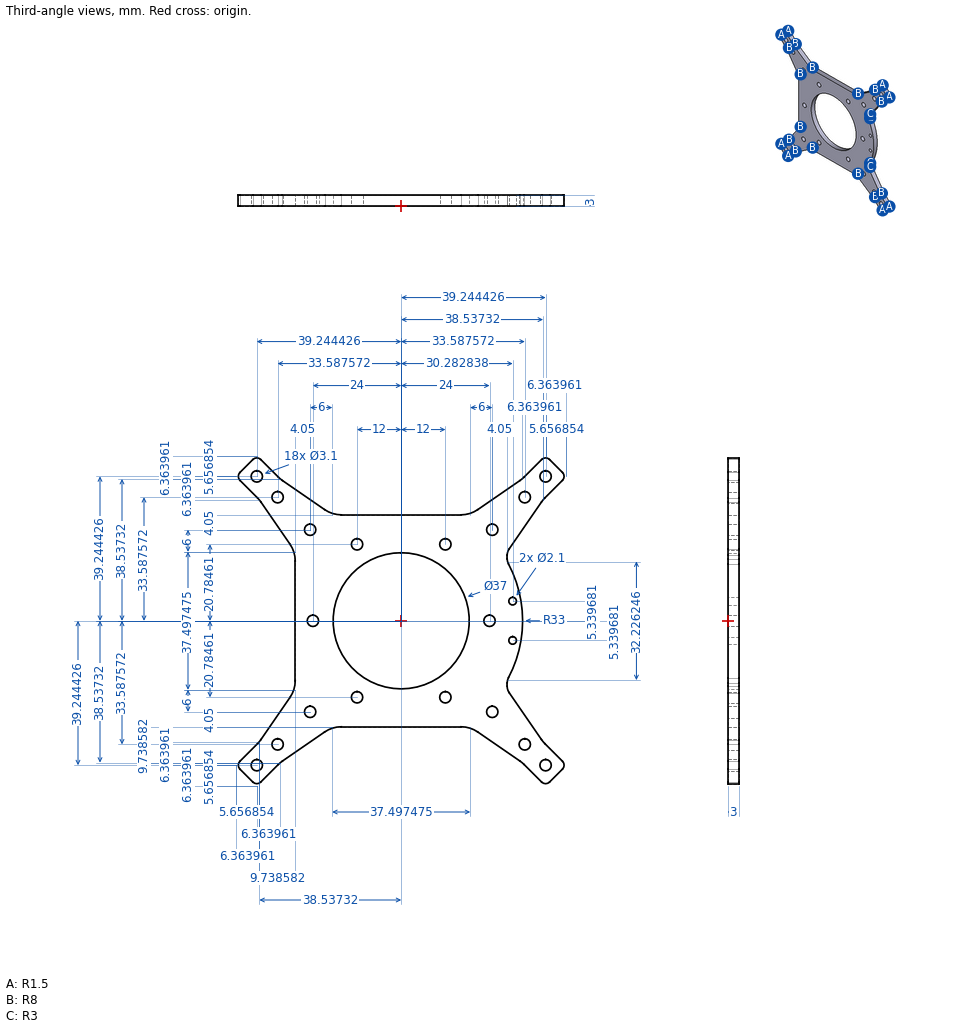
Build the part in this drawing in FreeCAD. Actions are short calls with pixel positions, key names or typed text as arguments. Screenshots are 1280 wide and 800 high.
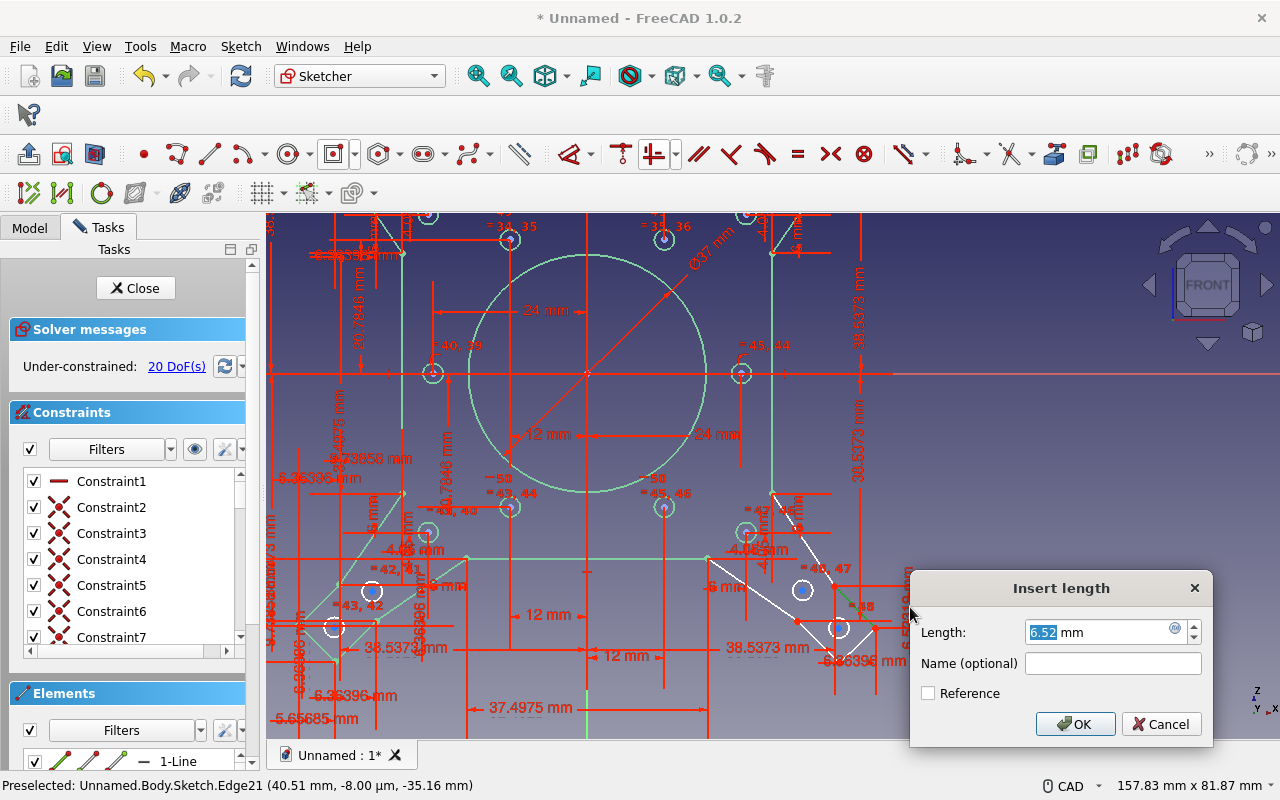
text(6.363961)
key(Return)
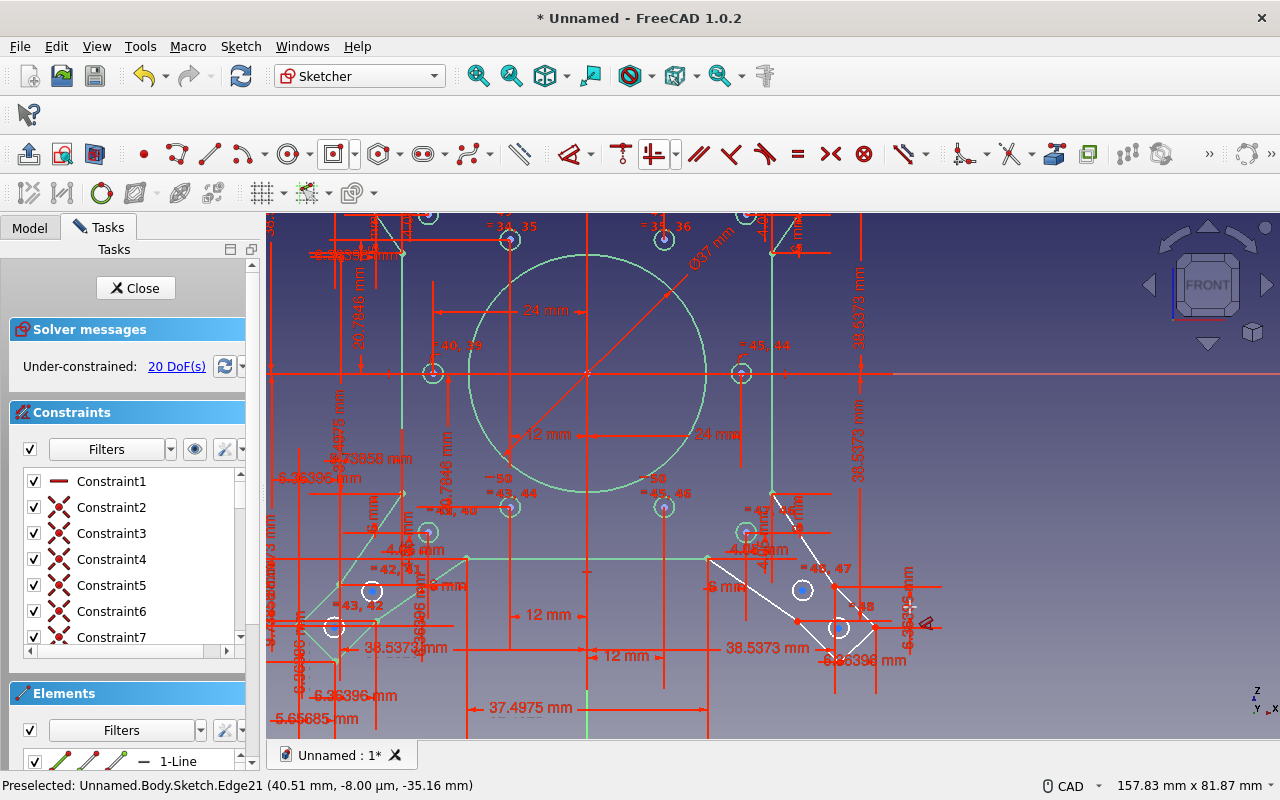
click(865, 638)
click(858, 697)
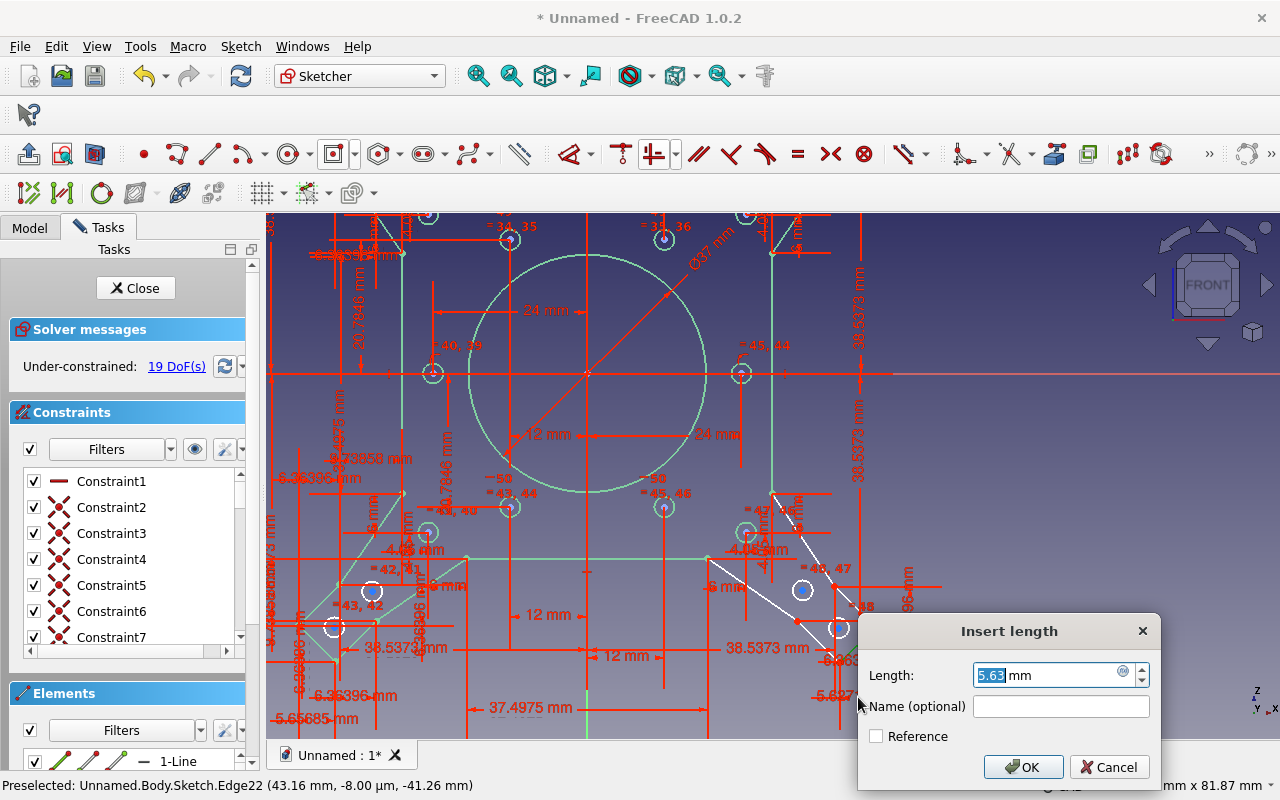
text(5.656854)
key(Return)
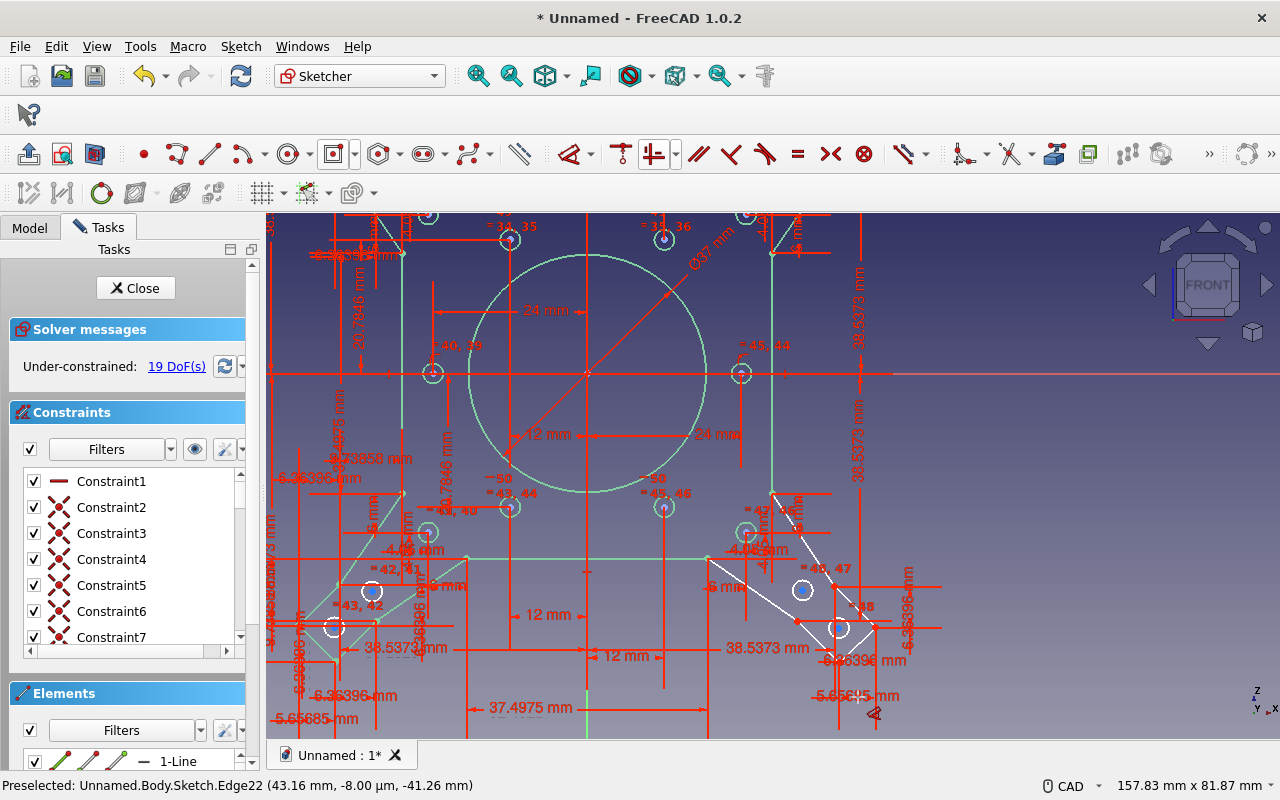
click(865, 638)
click(910, 637)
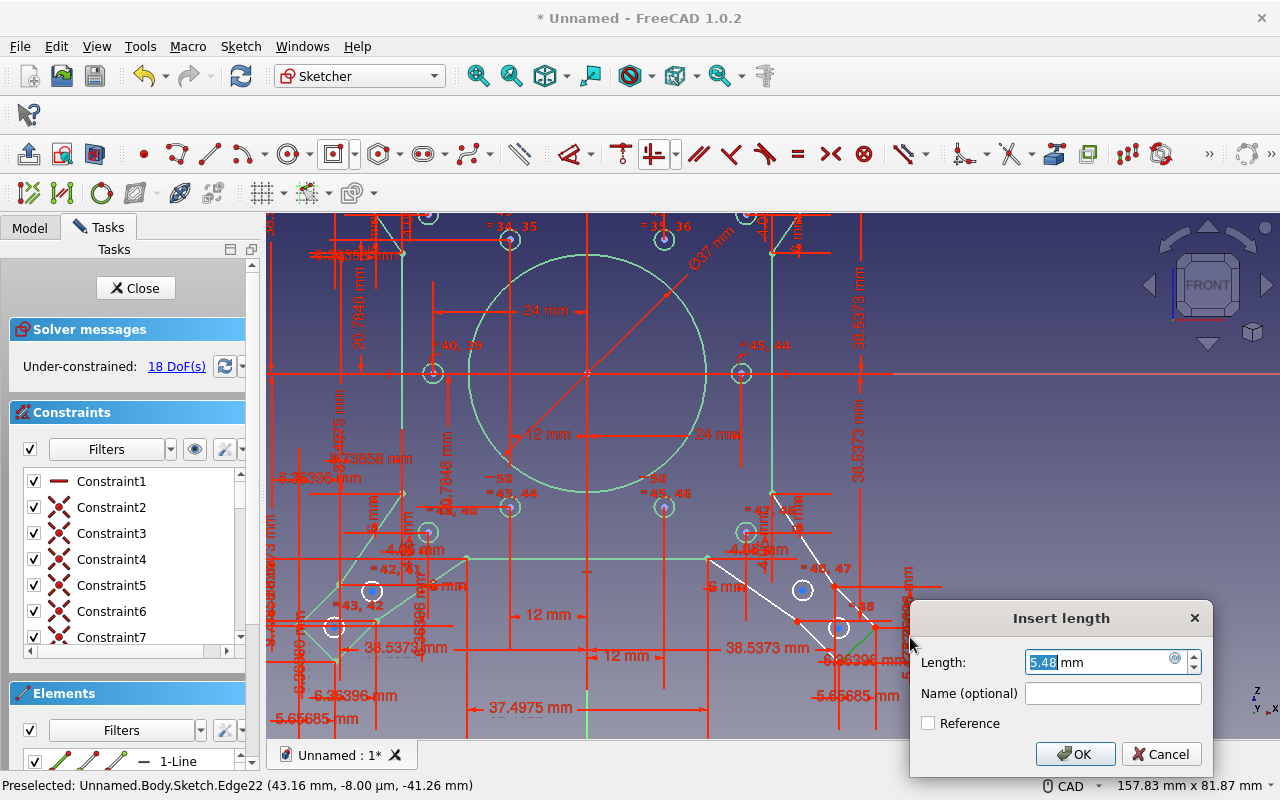
text(5.656854)
key(Return)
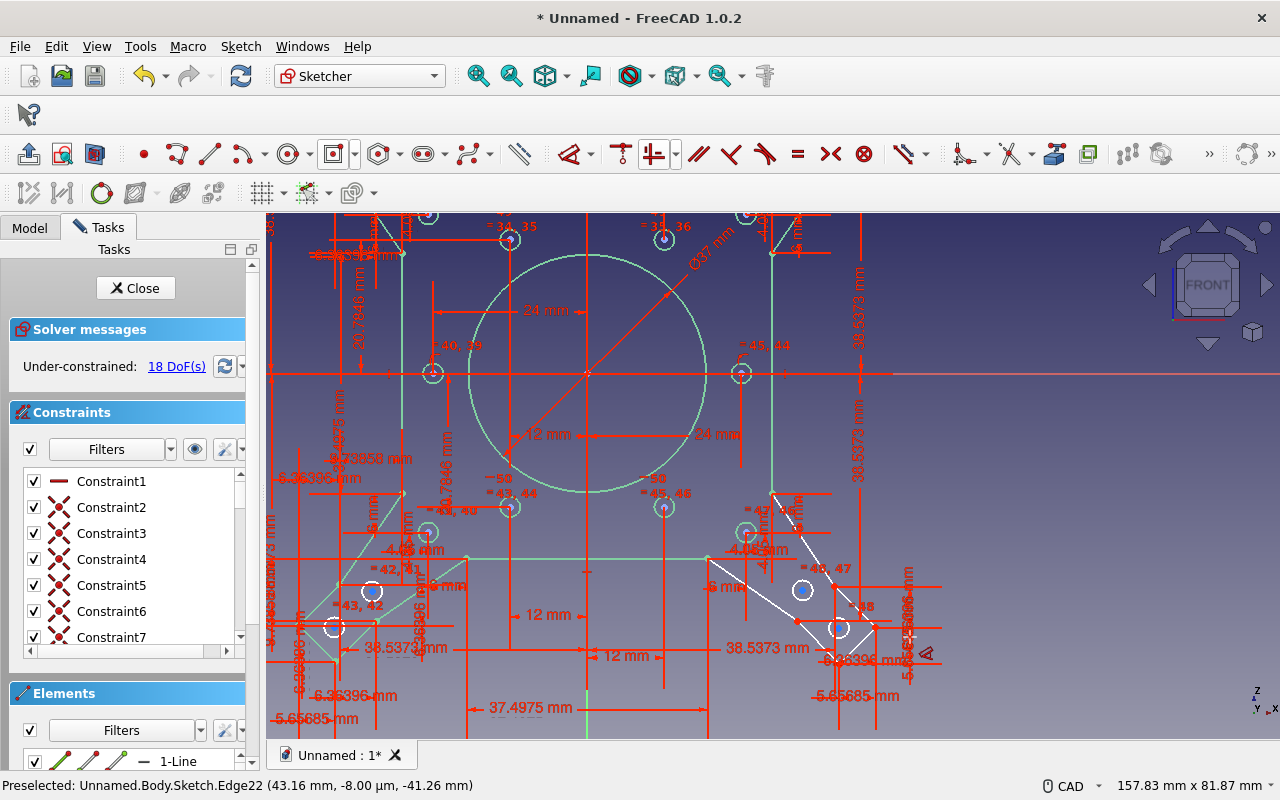
click(827, 651)
click(819, 491)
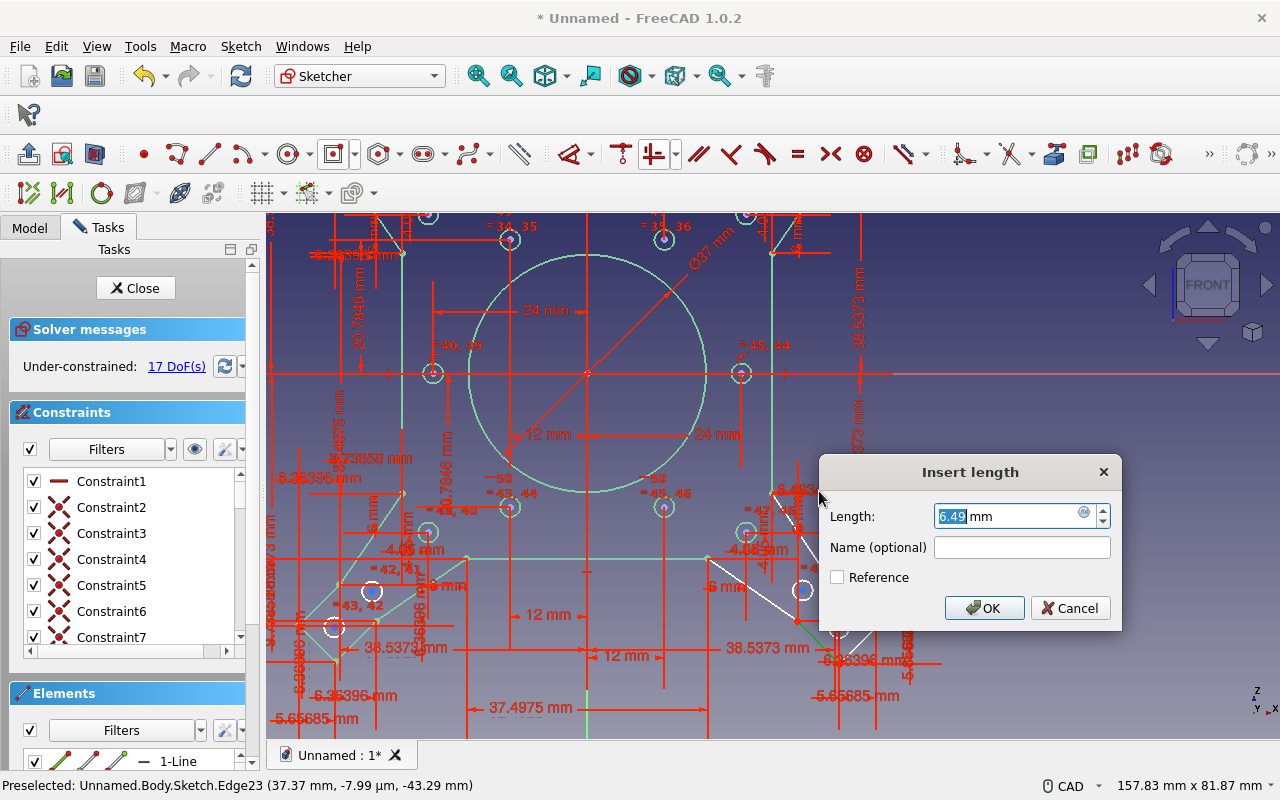
text(6.363961)
key(Return)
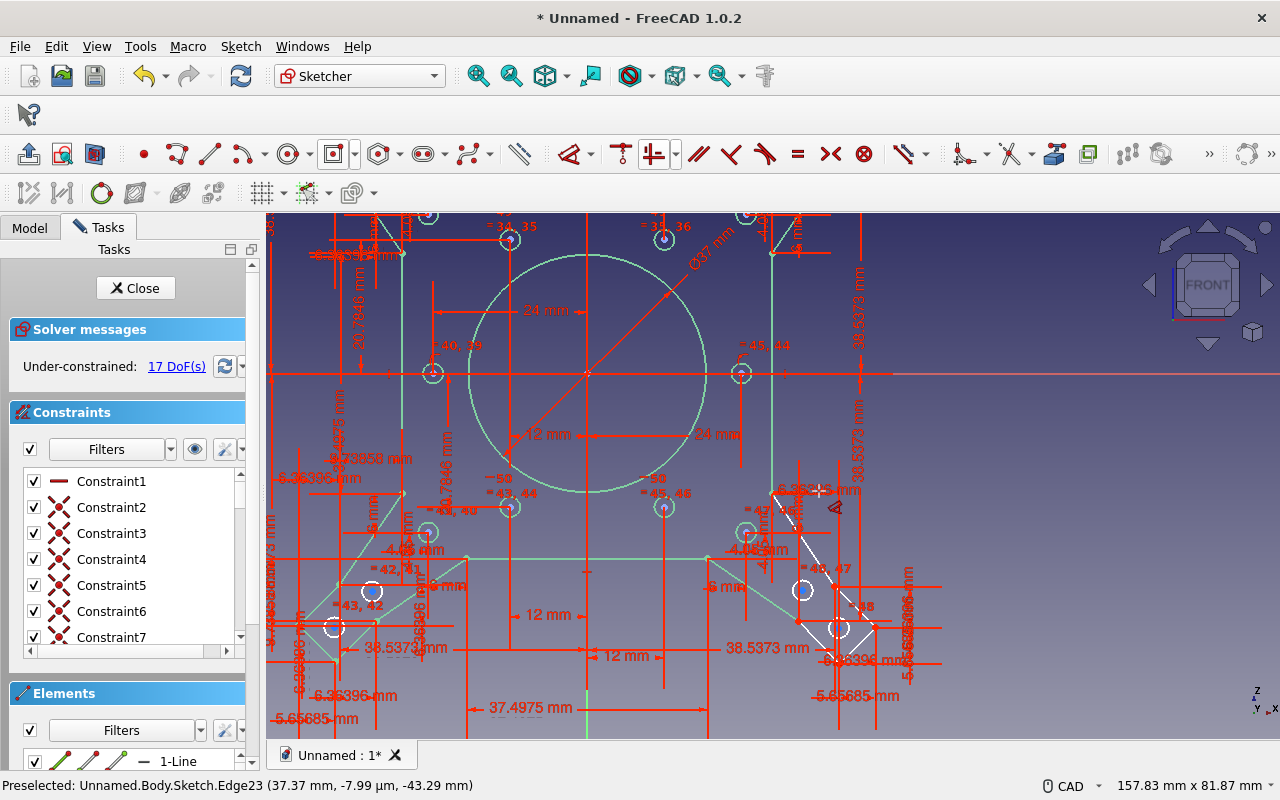
click(827, 651)
click(765, 628)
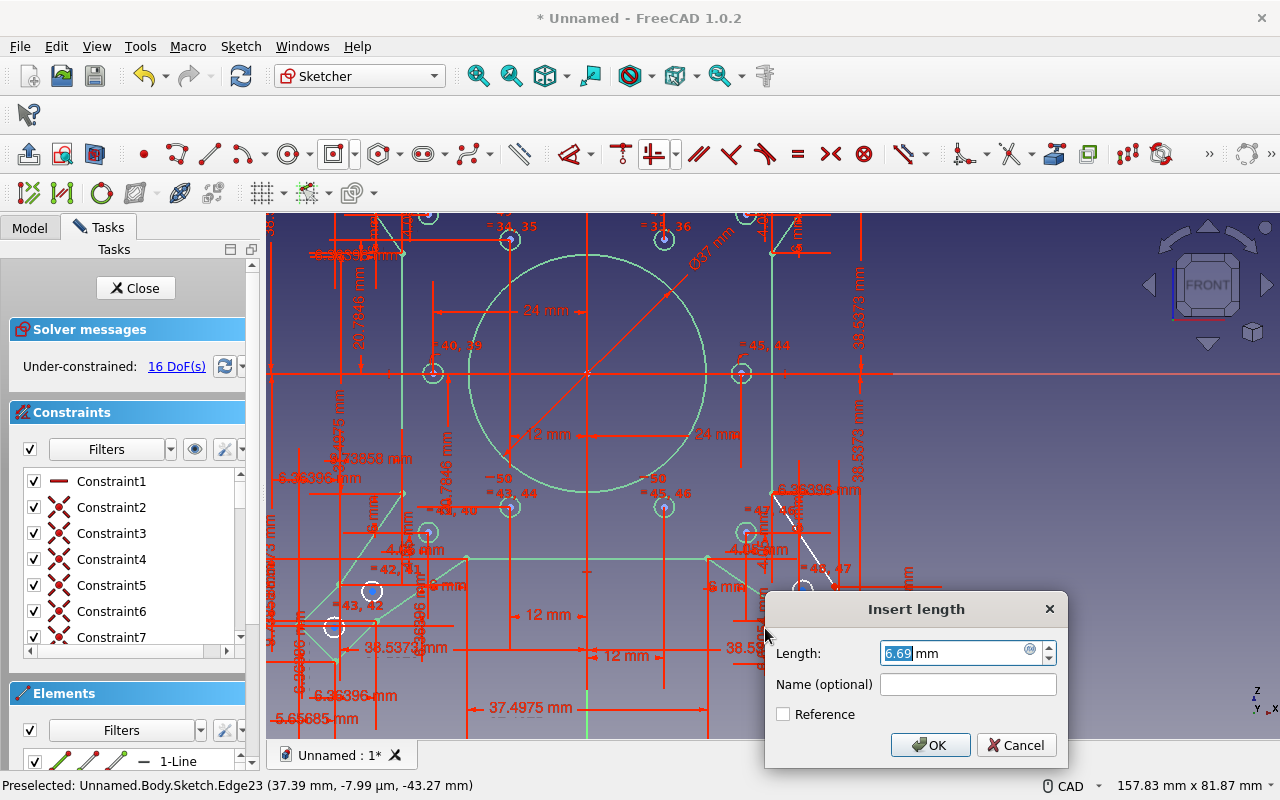
text(6.363961)
key(Return)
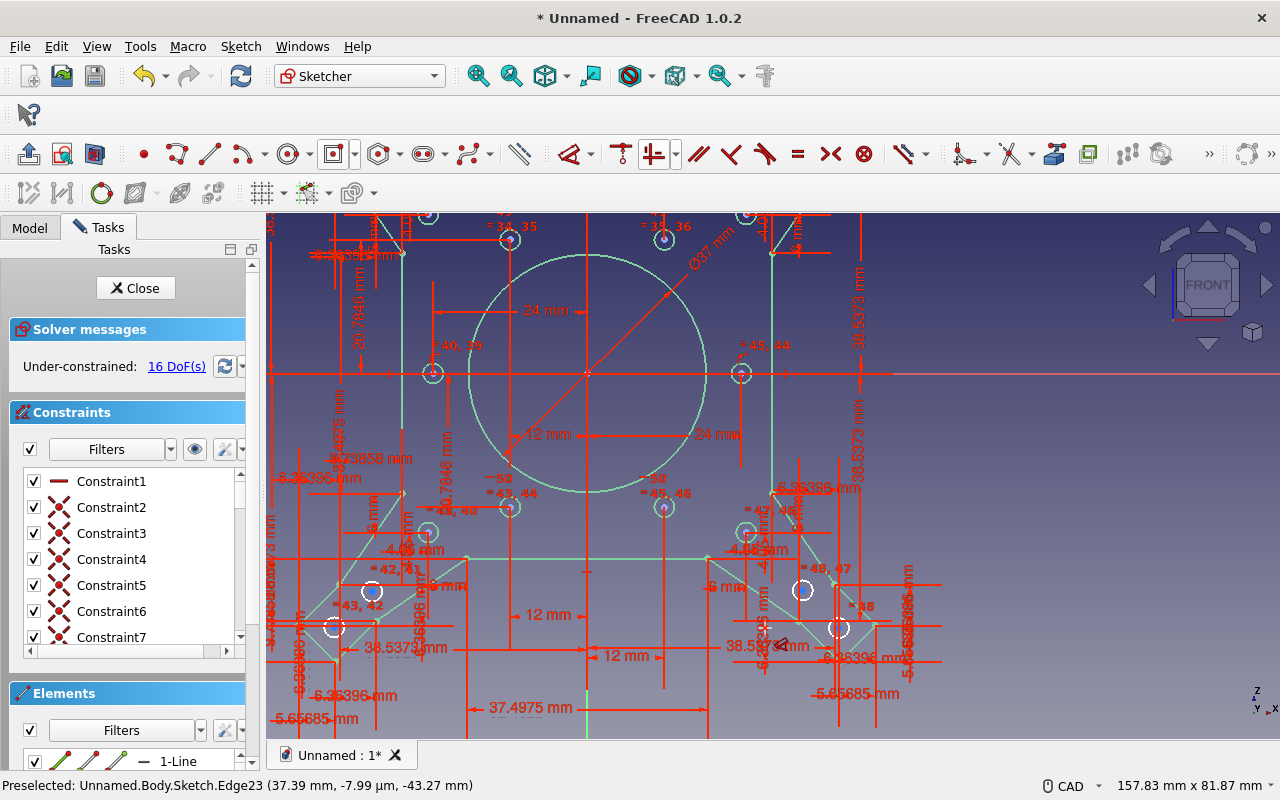
scroll(847, 601, down, 3)